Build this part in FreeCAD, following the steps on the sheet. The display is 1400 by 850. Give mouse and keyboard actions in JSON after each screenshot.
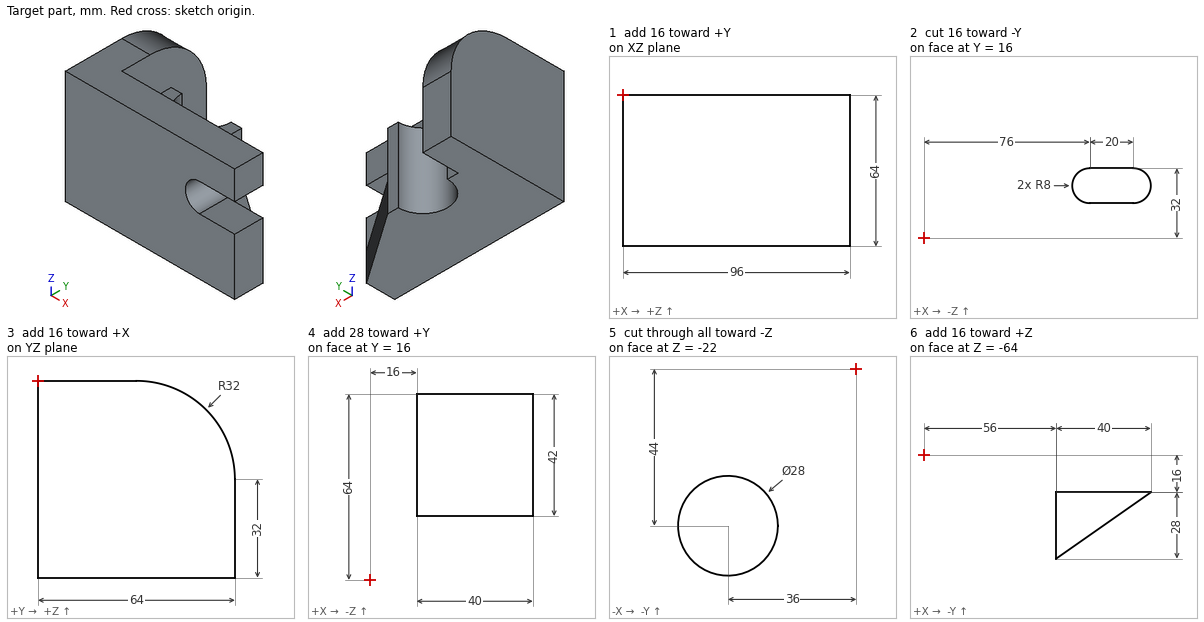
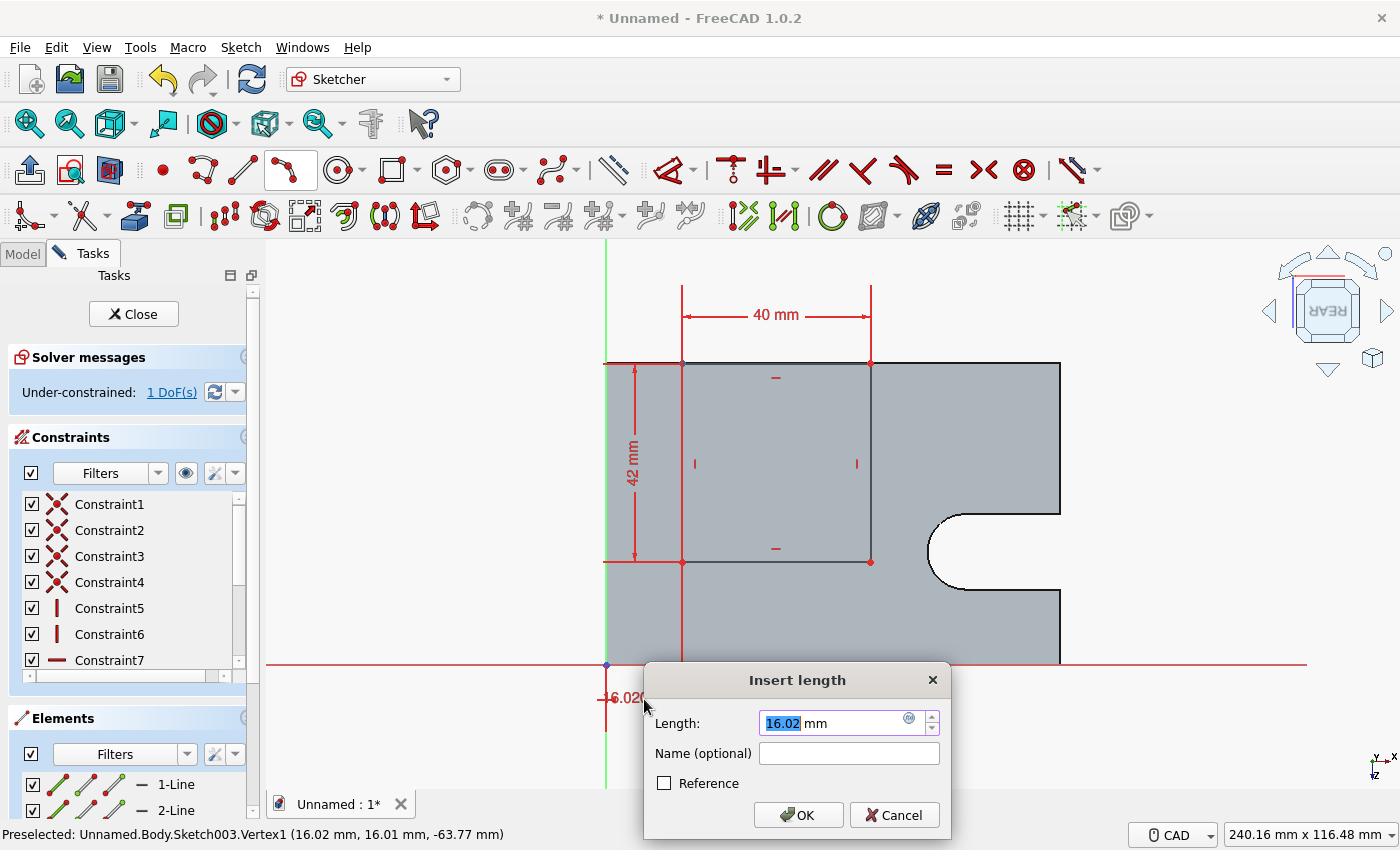
{"action": "type", "text": "16"}
{"action": "key", "text": "Return"}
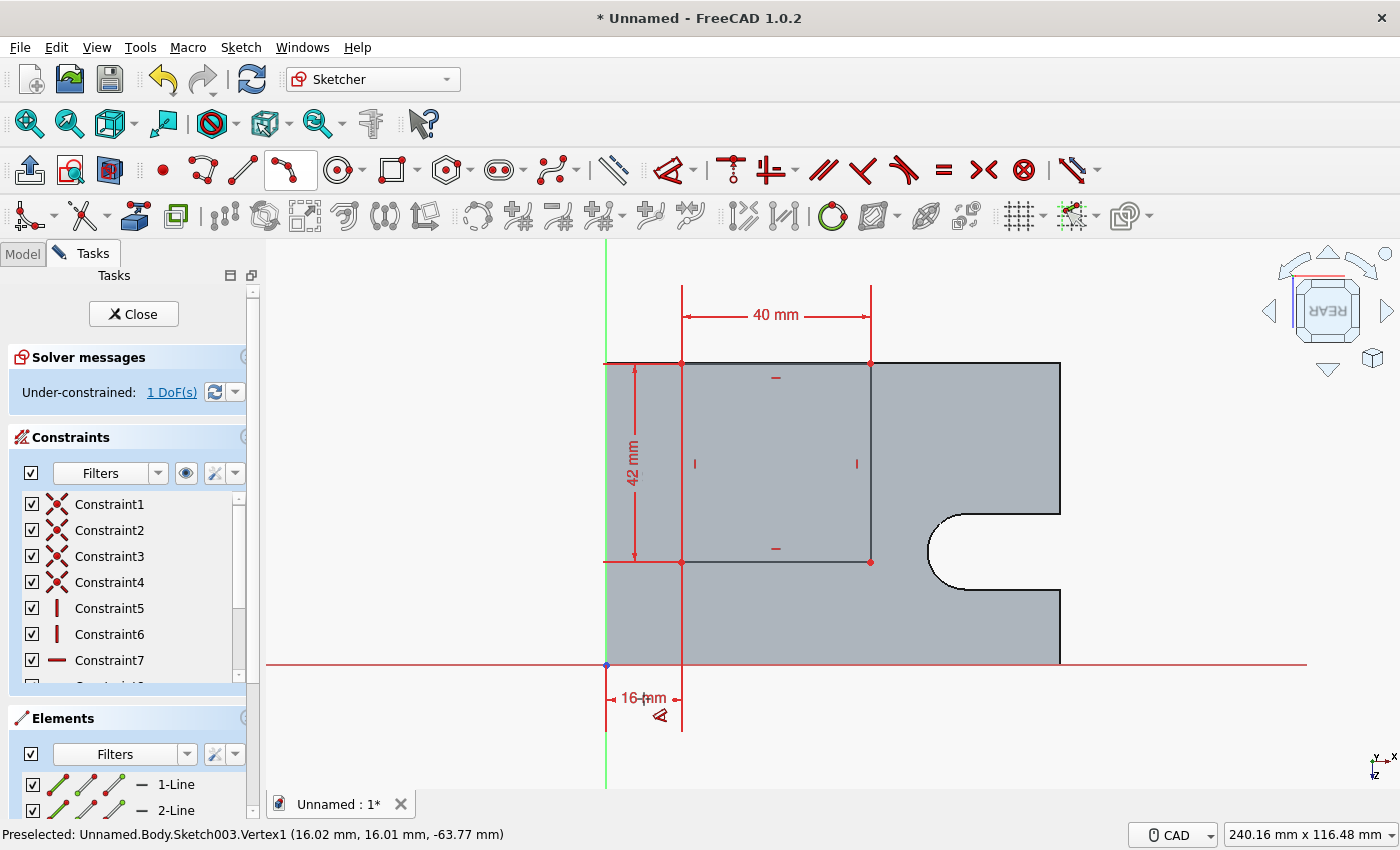
{"action": "left_click", "coordinate": [682, 364]}
{"action": "left_click", "coordinate": [572, 515]}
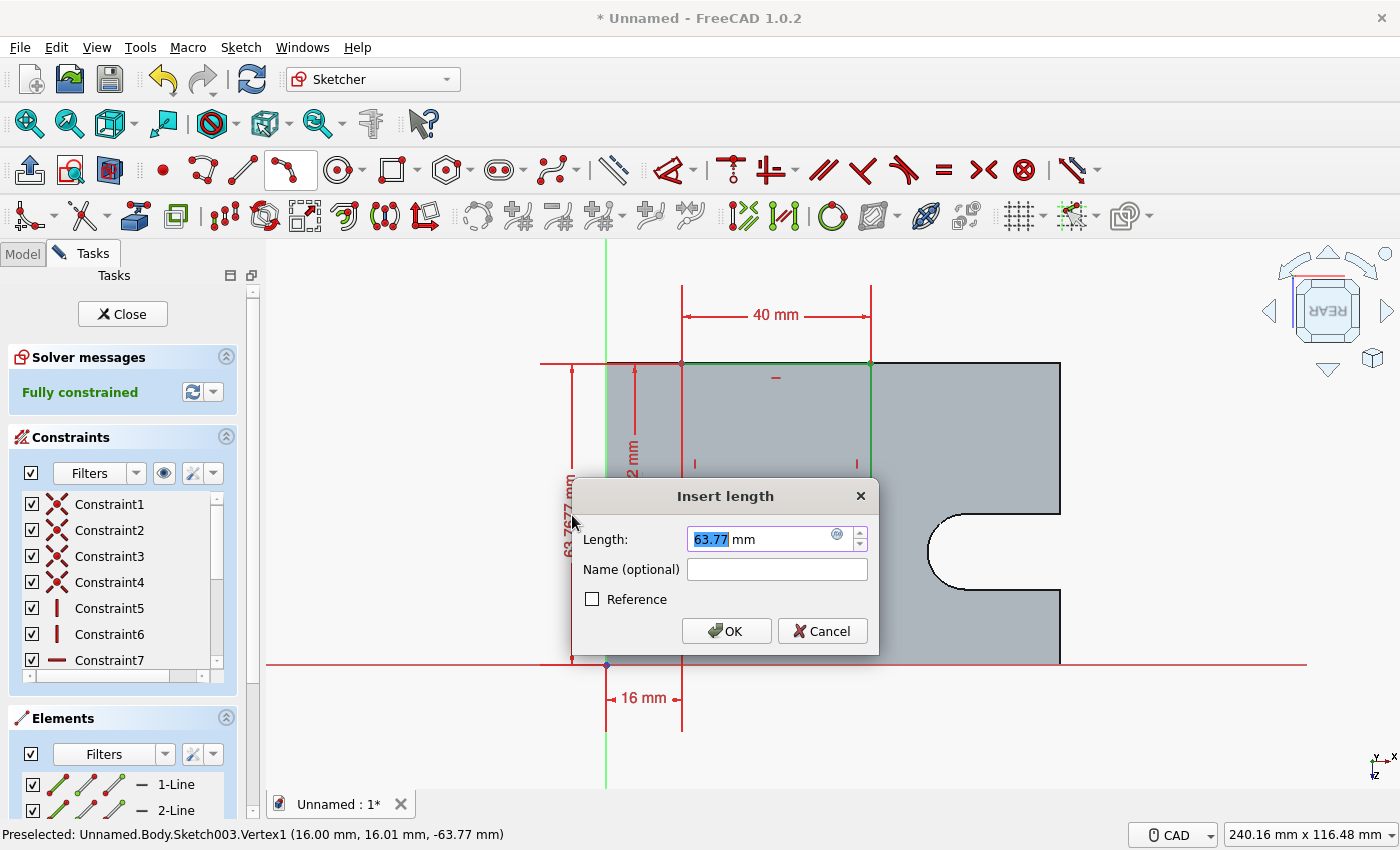
{"action": "type", "text": "64"}
{"action": "key", "text": "Return"}
{"action": "key", "text": "Escape"}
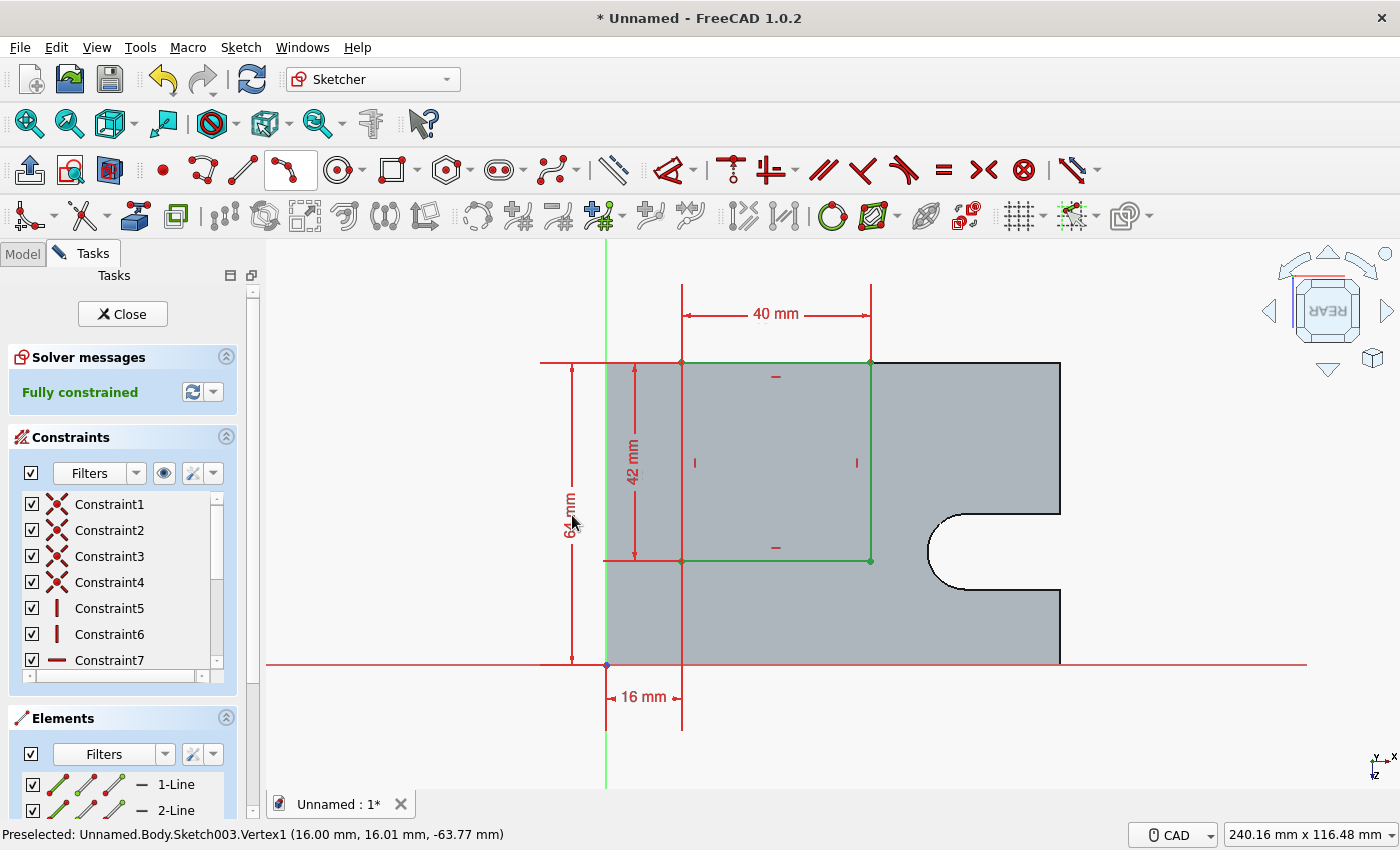
{"action": "left_click", "coordinate": [123, 314]}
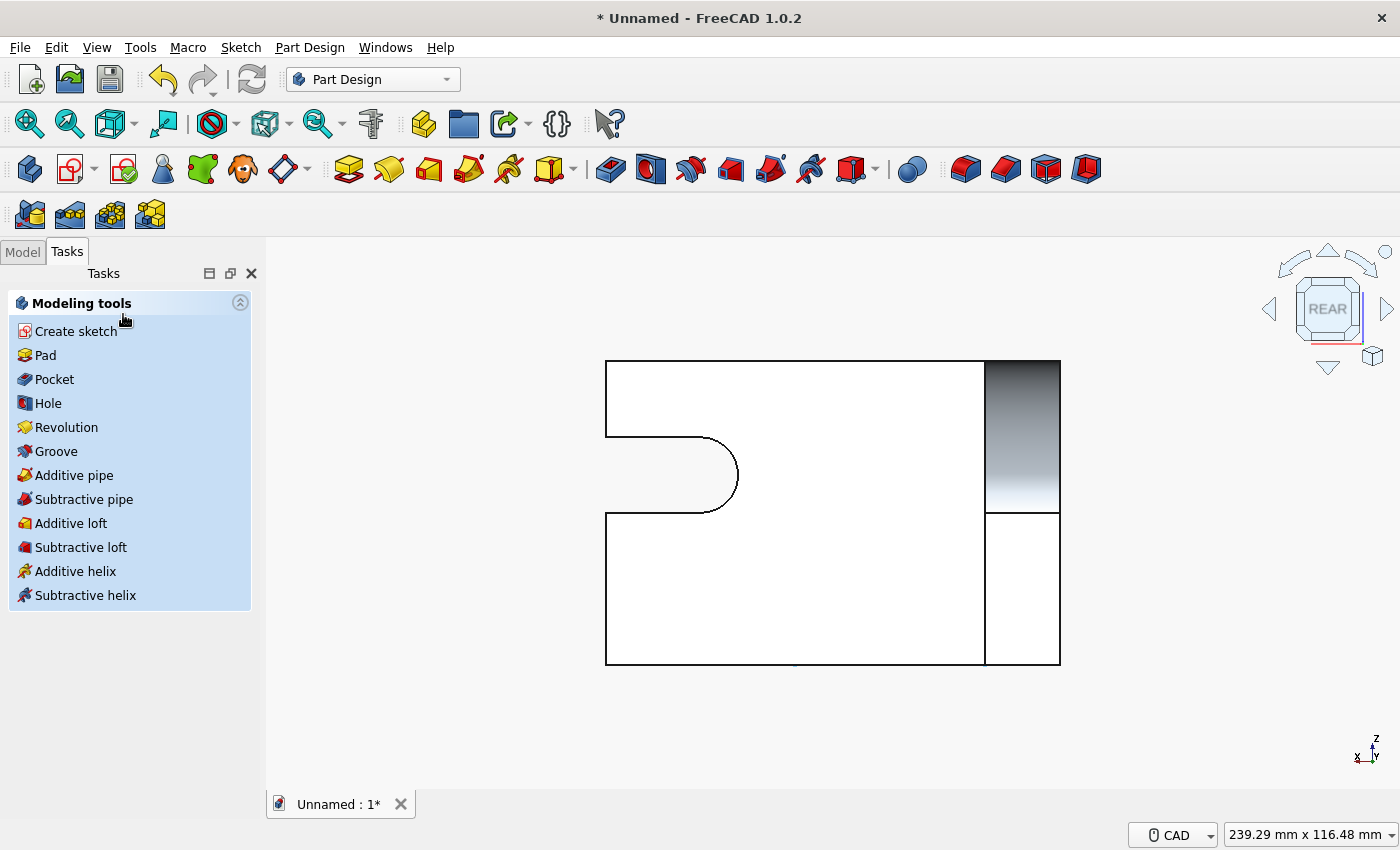
{"action": "left_click", "coordinate": [350, 170]}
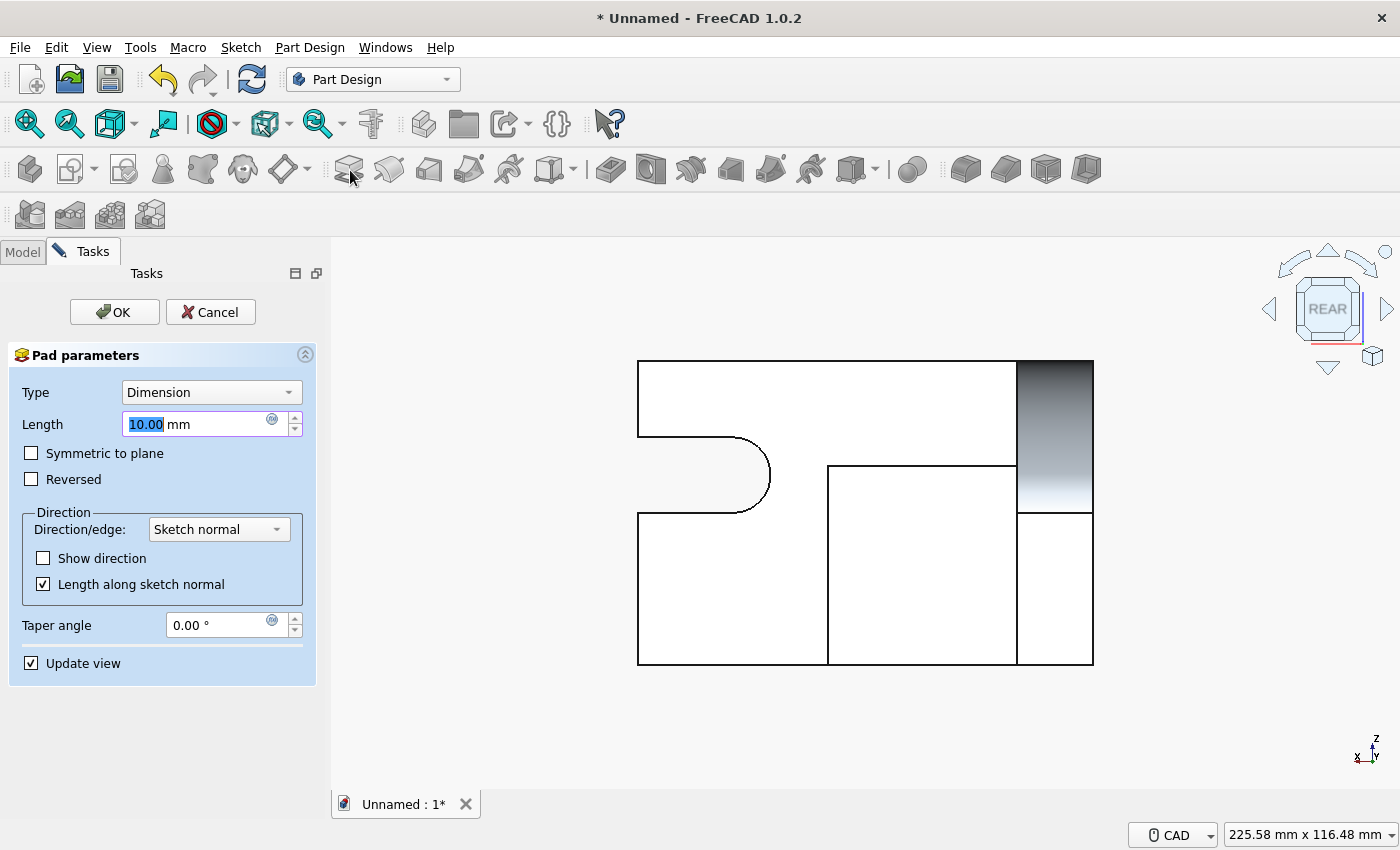
{"action": "type", "text": "28"}
{"action": "key", "text": "Tab"}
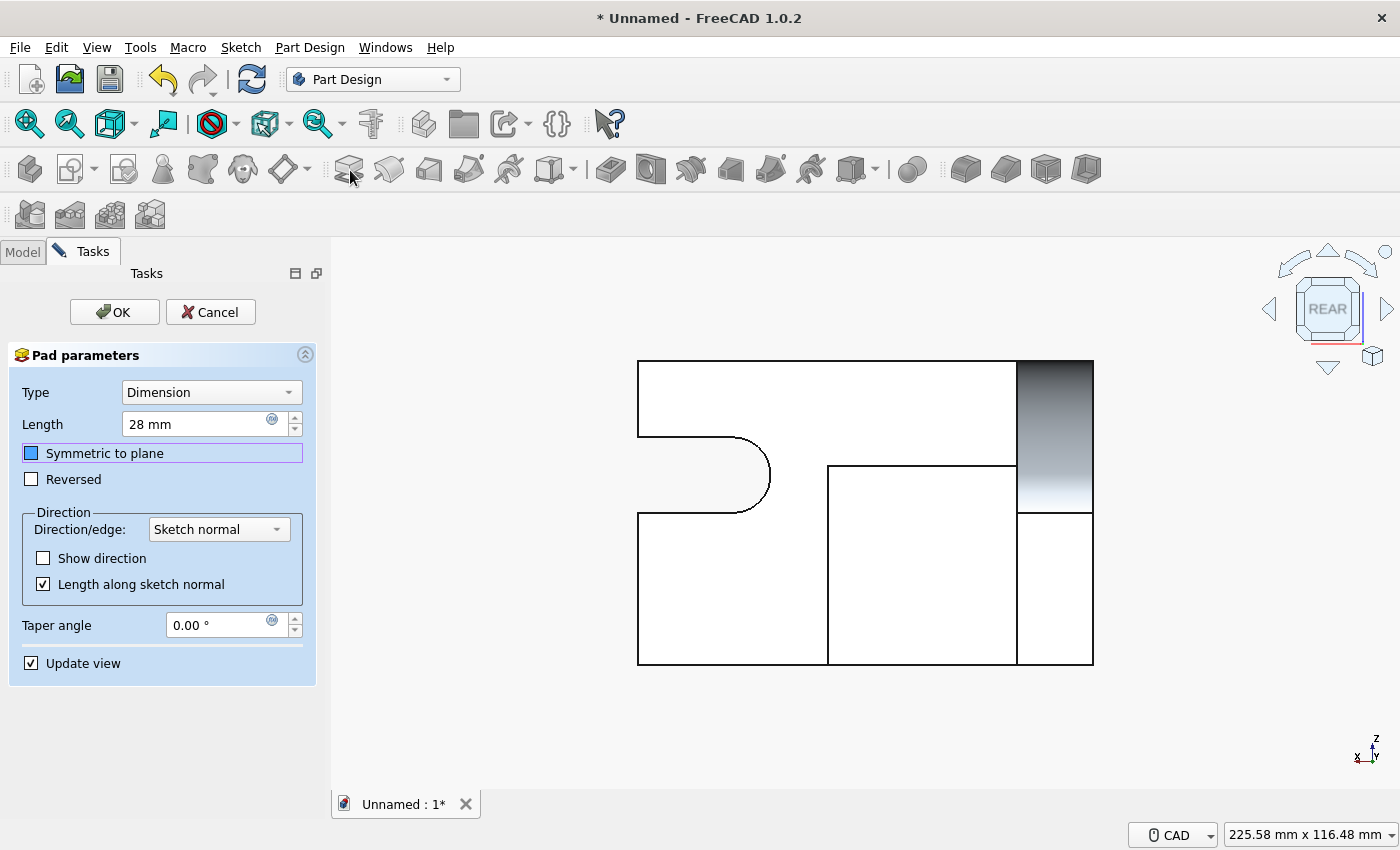
{"action": "left_click", "coordinate": [115, 312]}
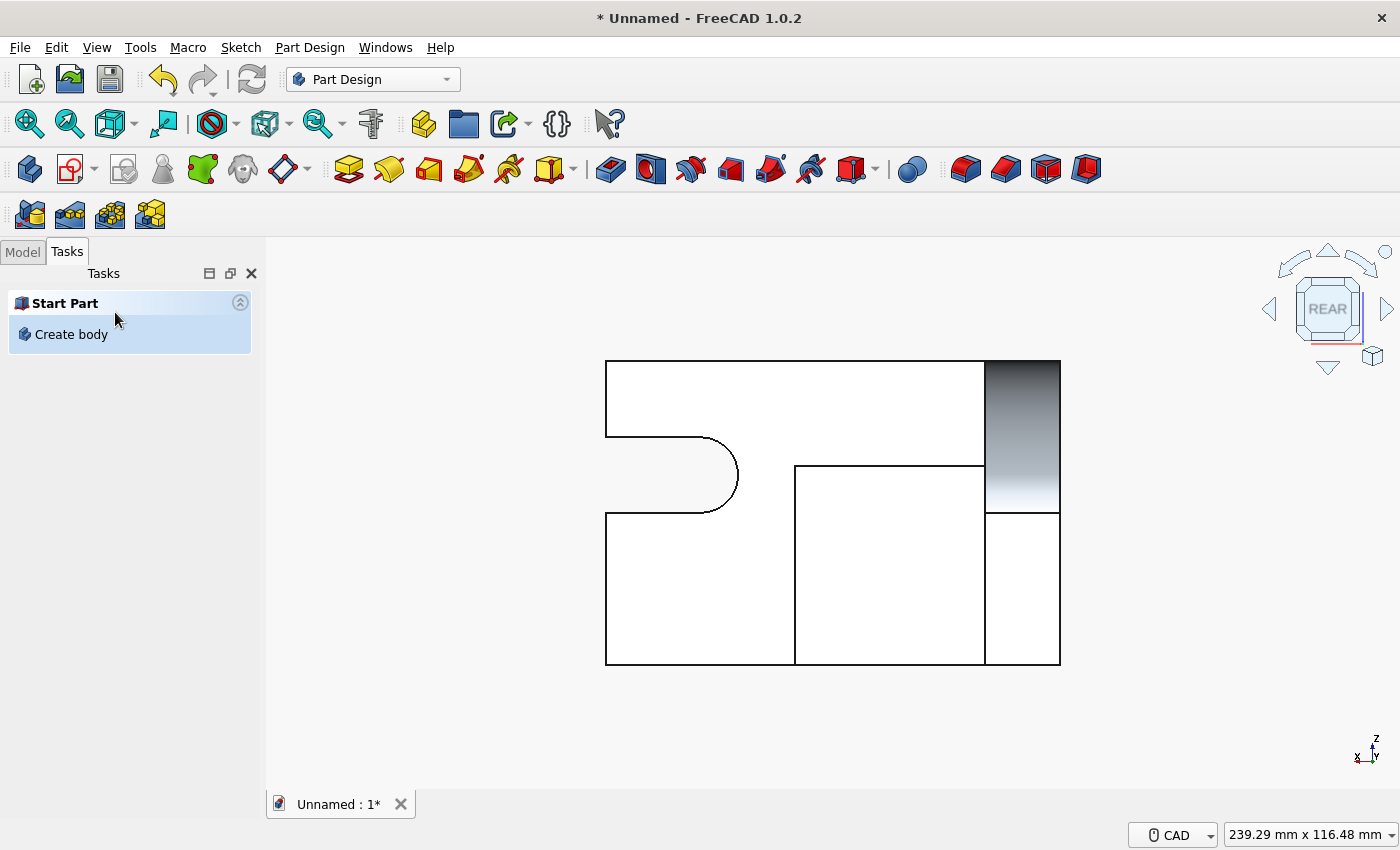
{"action": "key", "text": "0"}